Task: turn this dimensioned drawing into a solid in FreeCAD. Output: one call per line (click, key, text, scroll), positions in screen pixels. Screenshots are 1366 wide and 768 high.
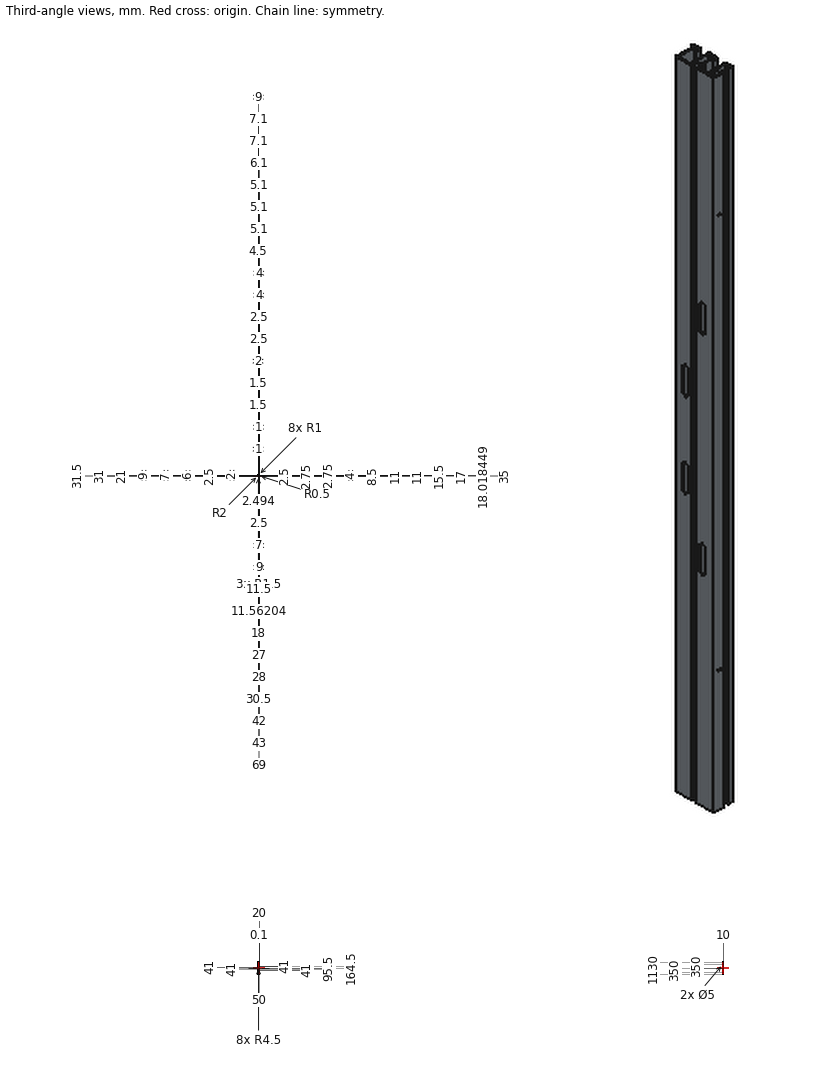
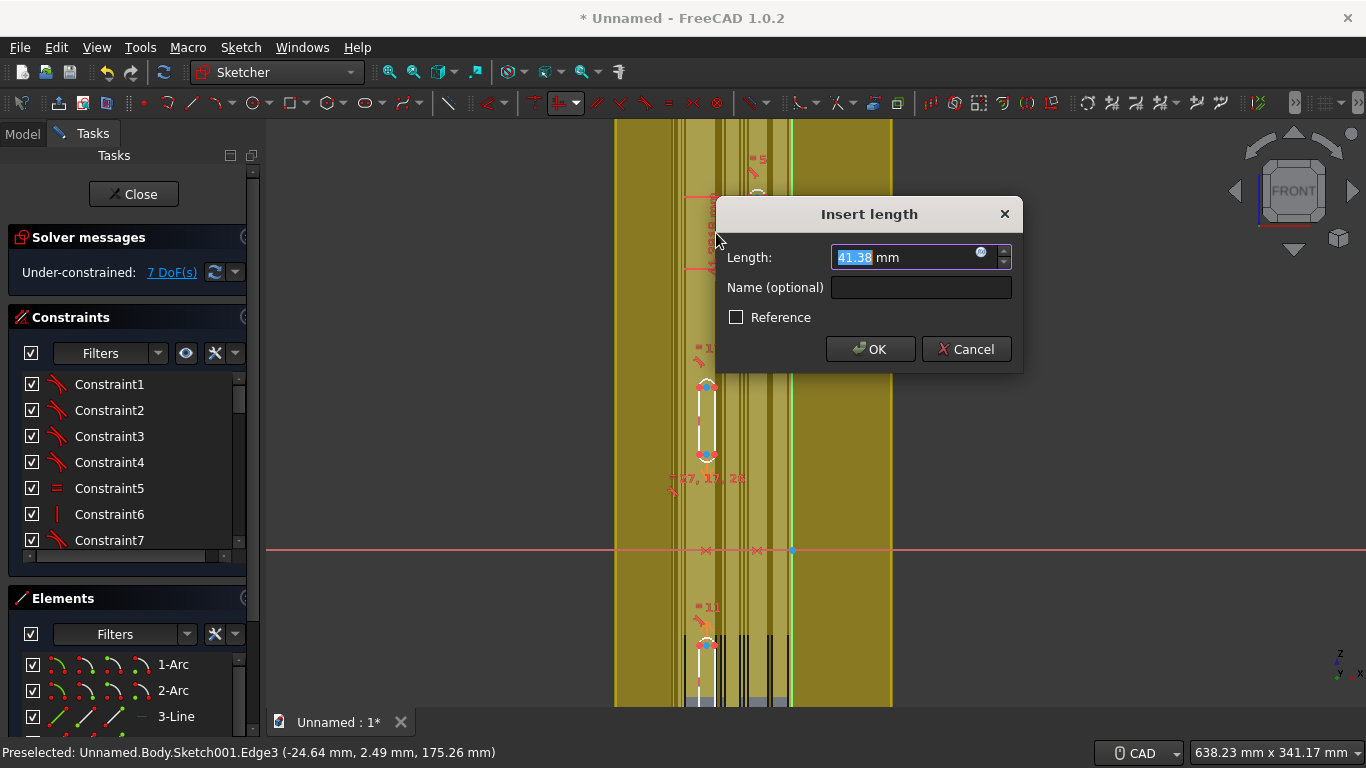
text(41)
key(Return)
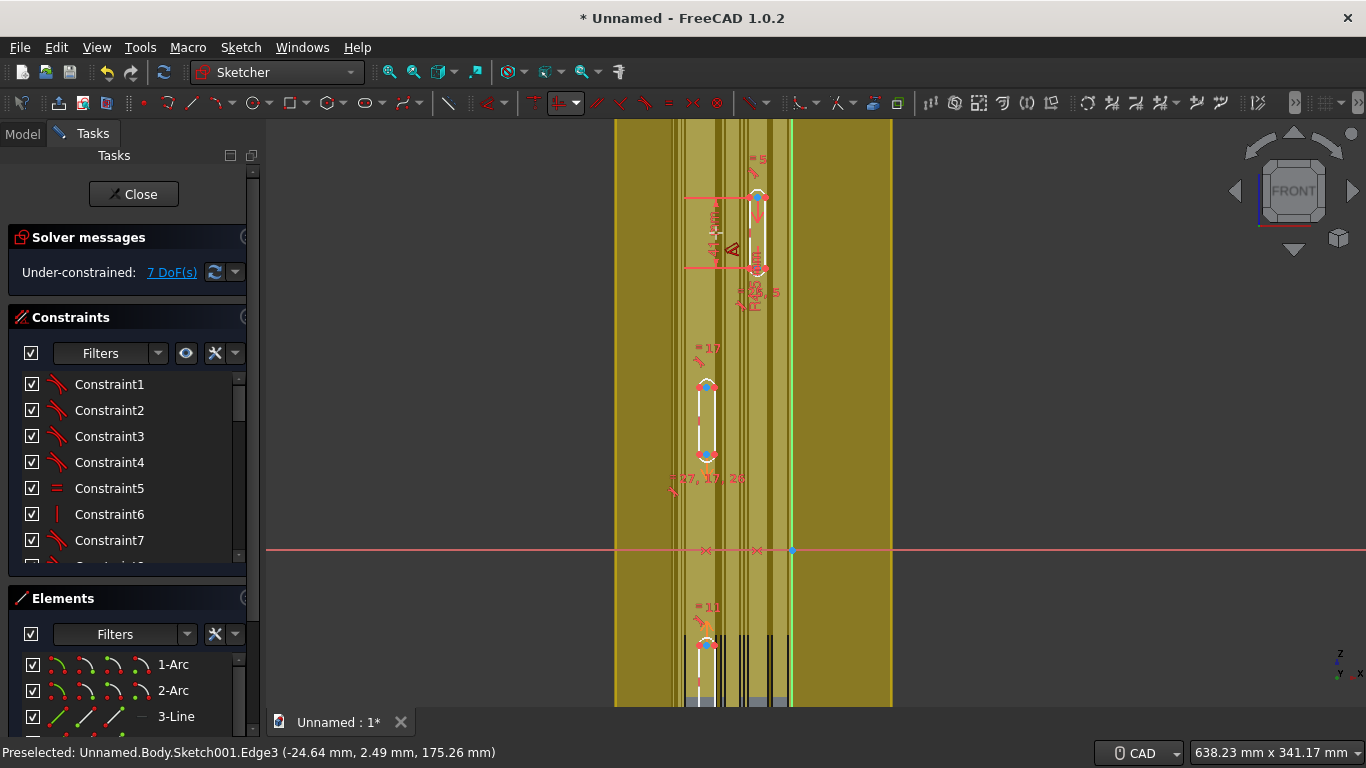
click(699, 667)
click(665, 662)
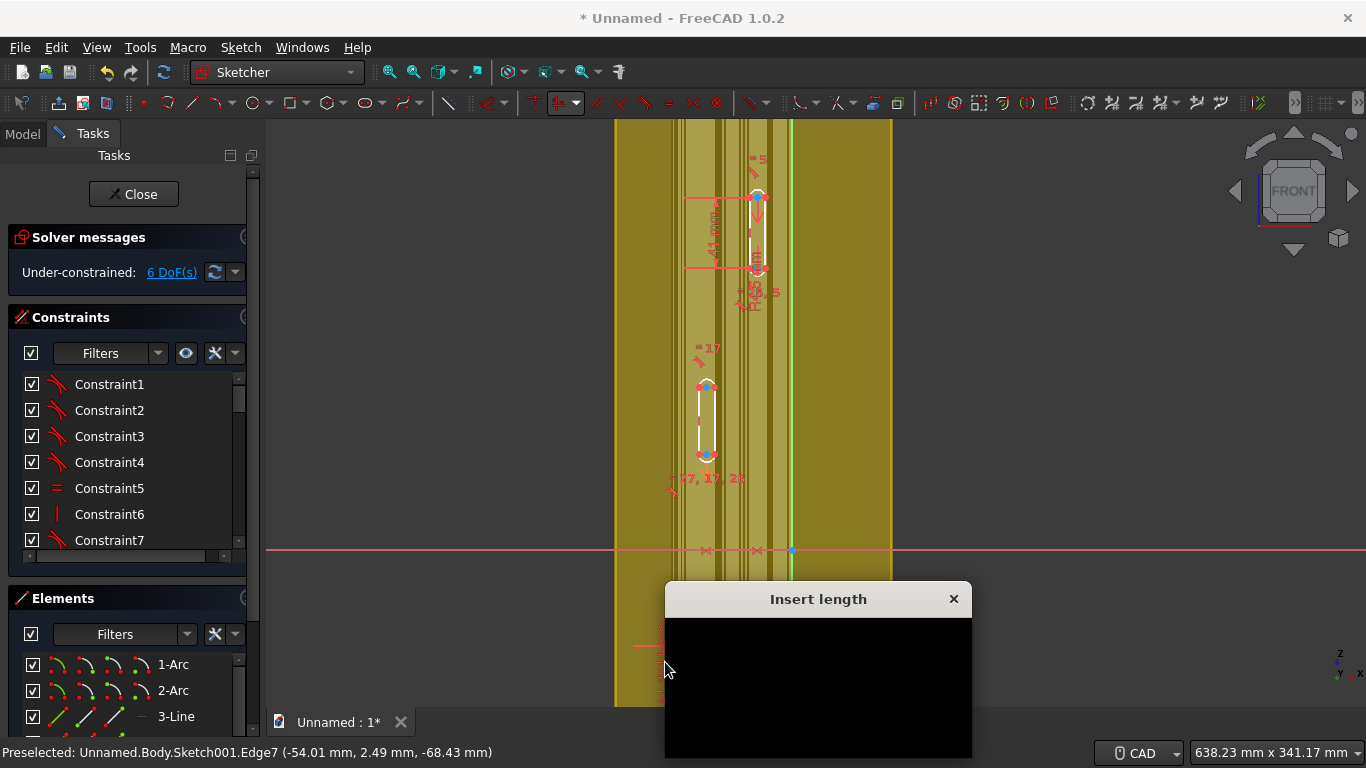
text(41)
key(Return)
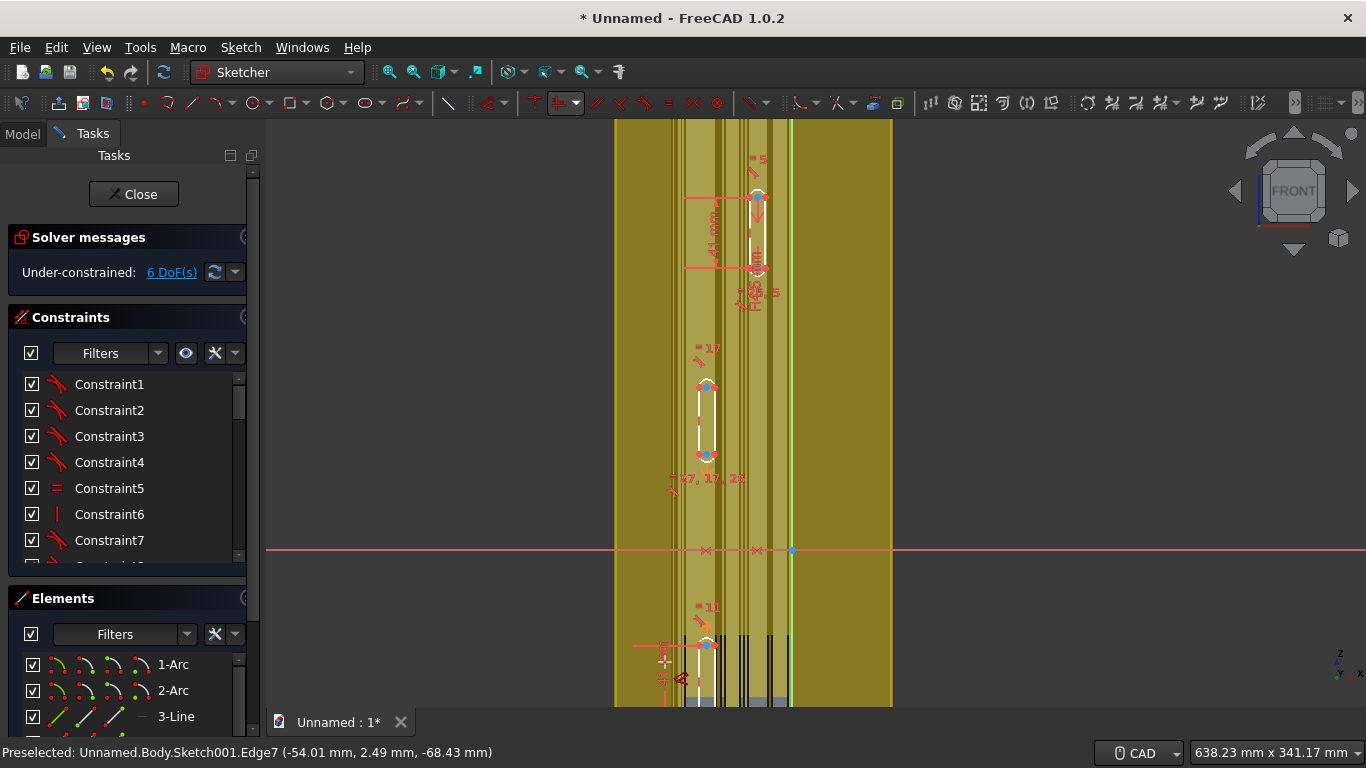
click(699, 434)
click(665, 421)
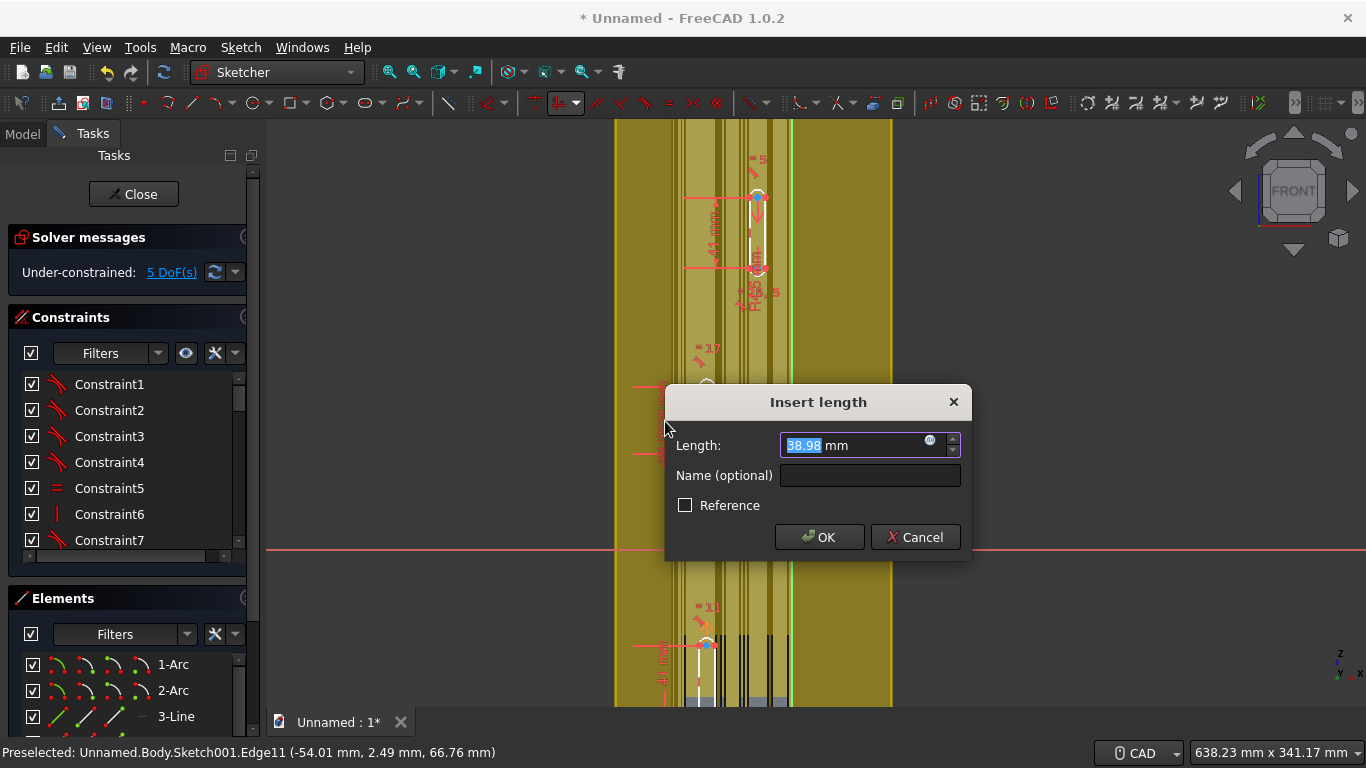
text(41)
key(Return)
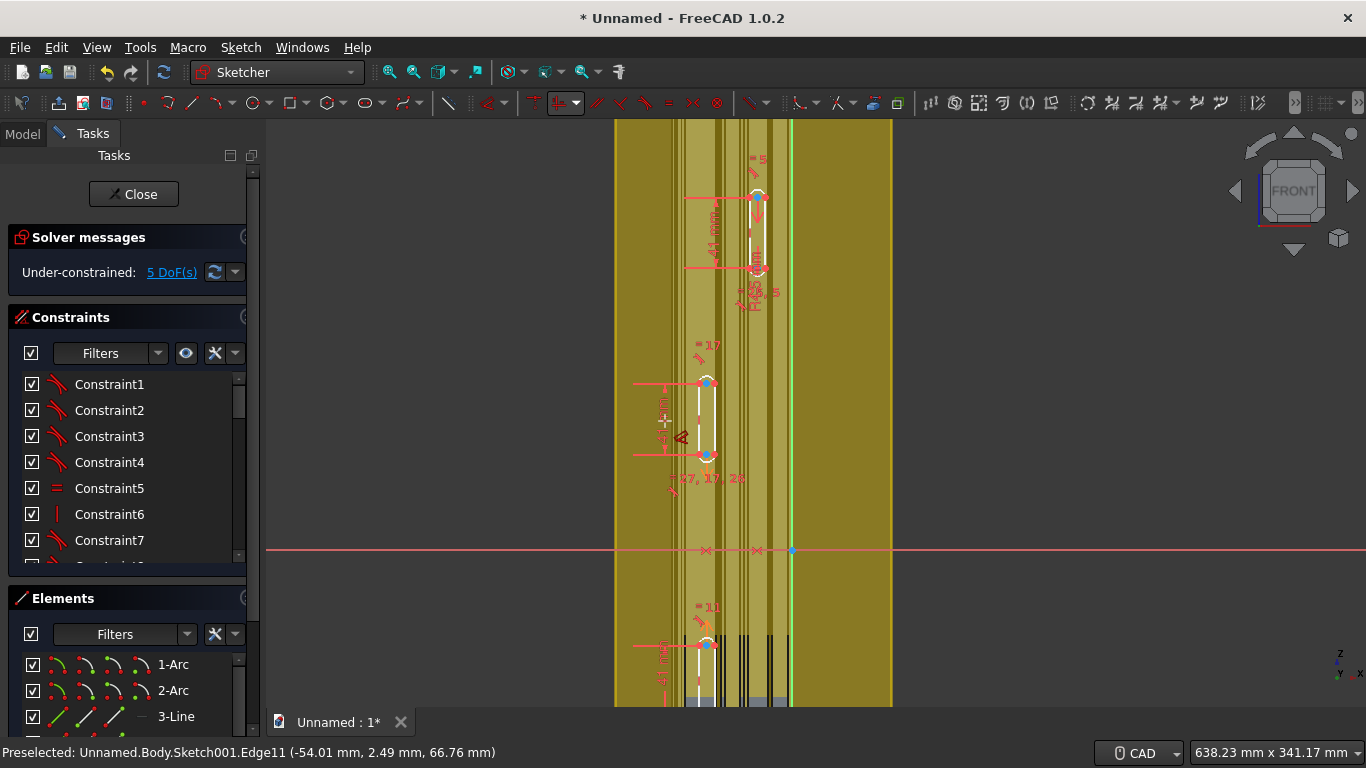
scroll(750, 246, down, 3)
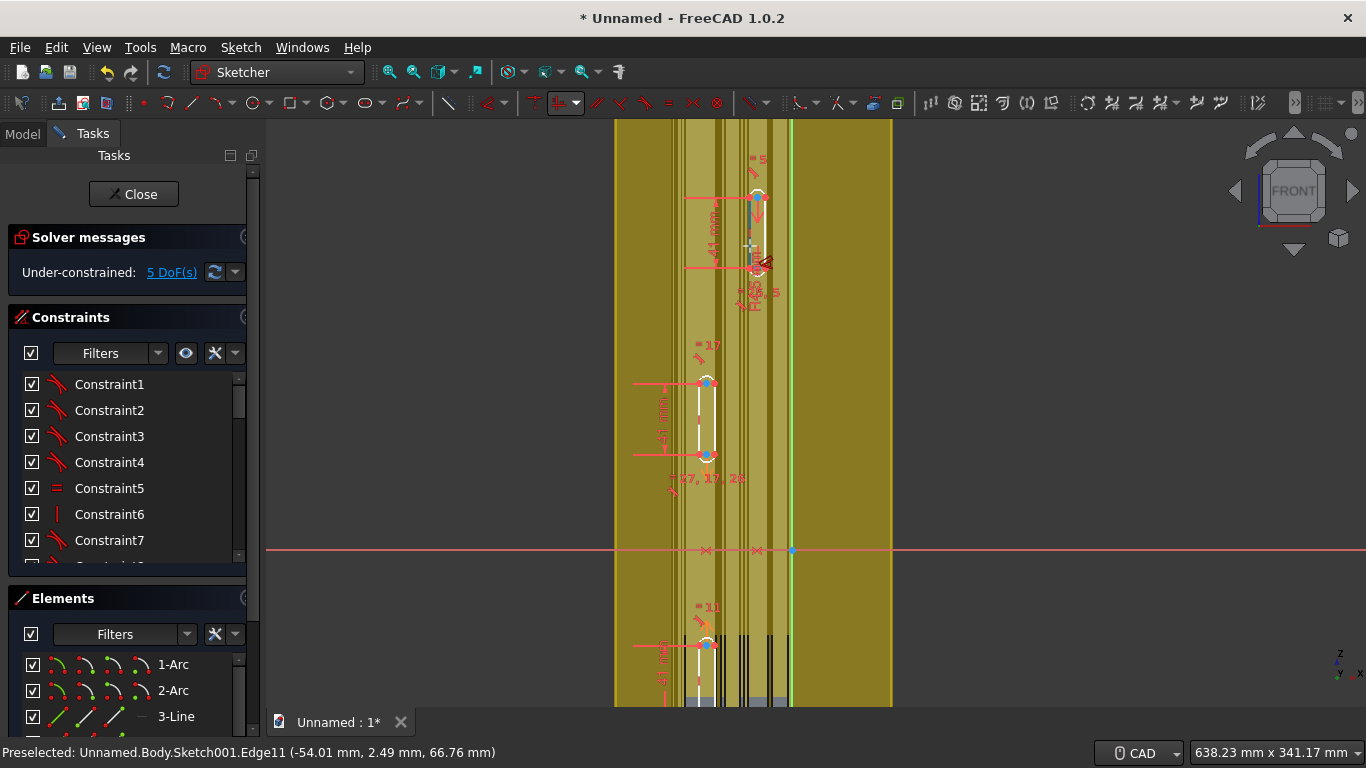
scroll(750, 595, up, 3)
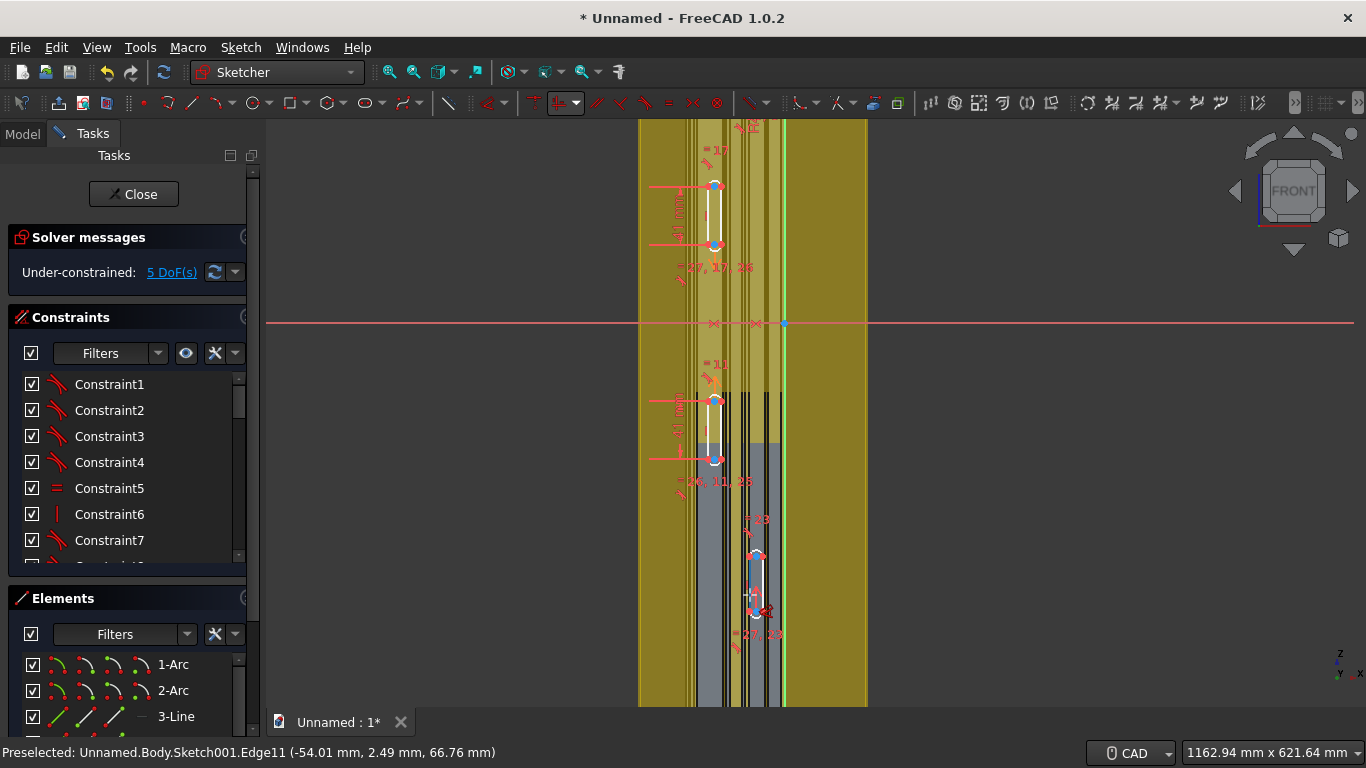
click(750, 595)
click(716, 582)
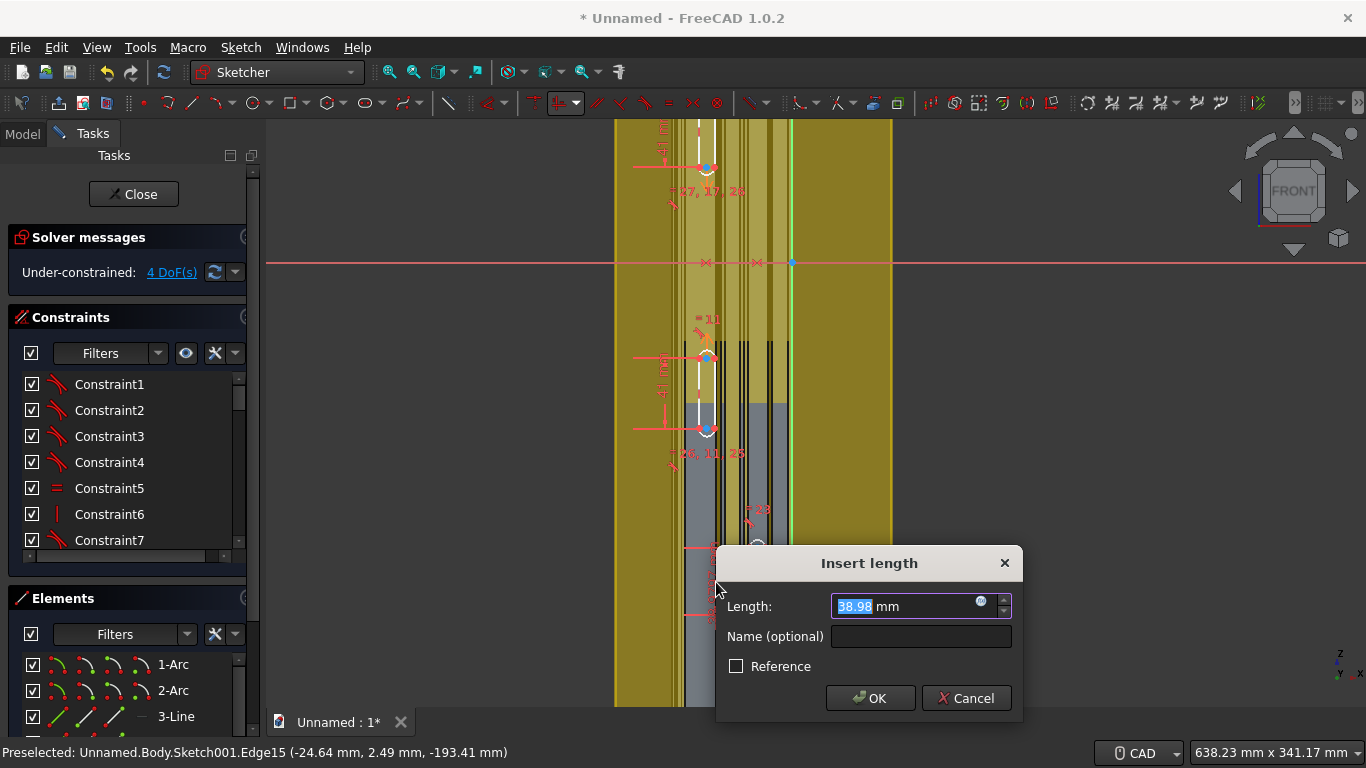
text(41)
key(Return)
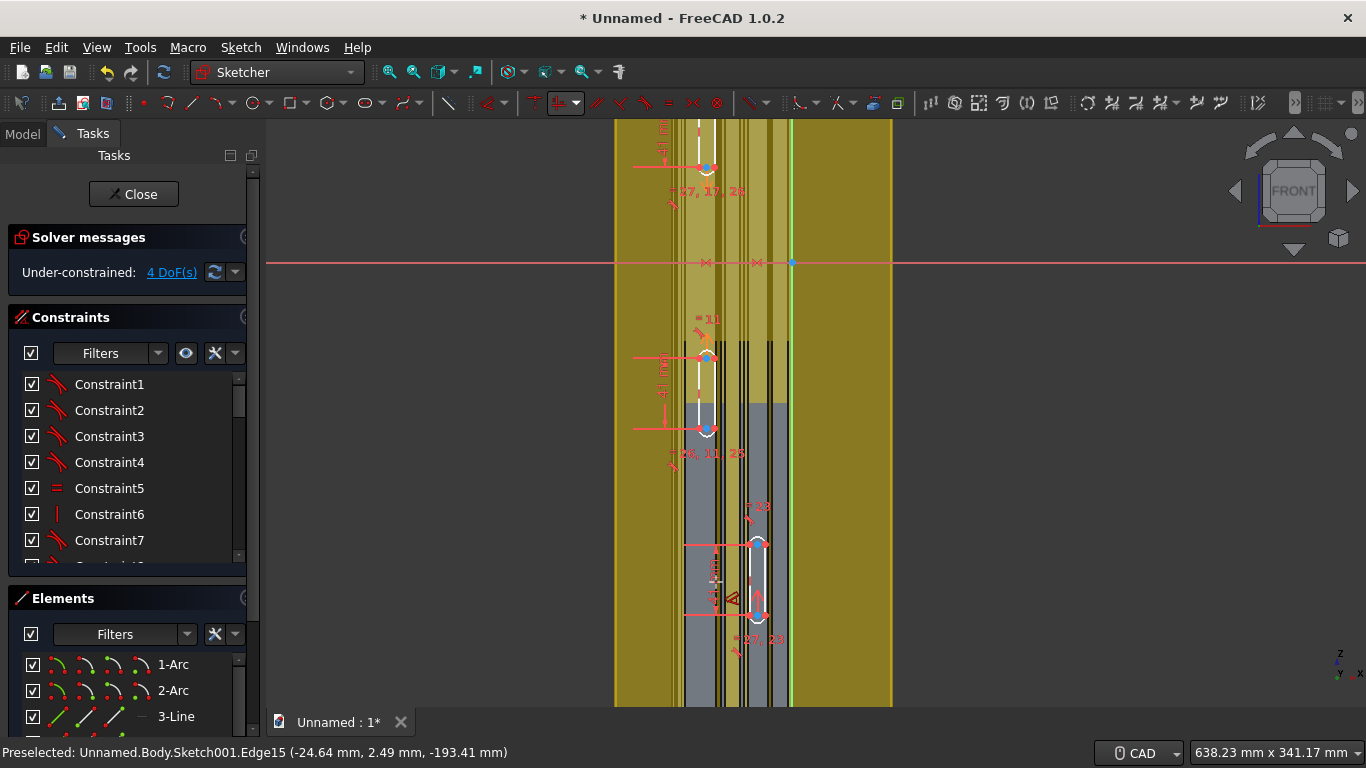
scroll(750, 596, down, 3)